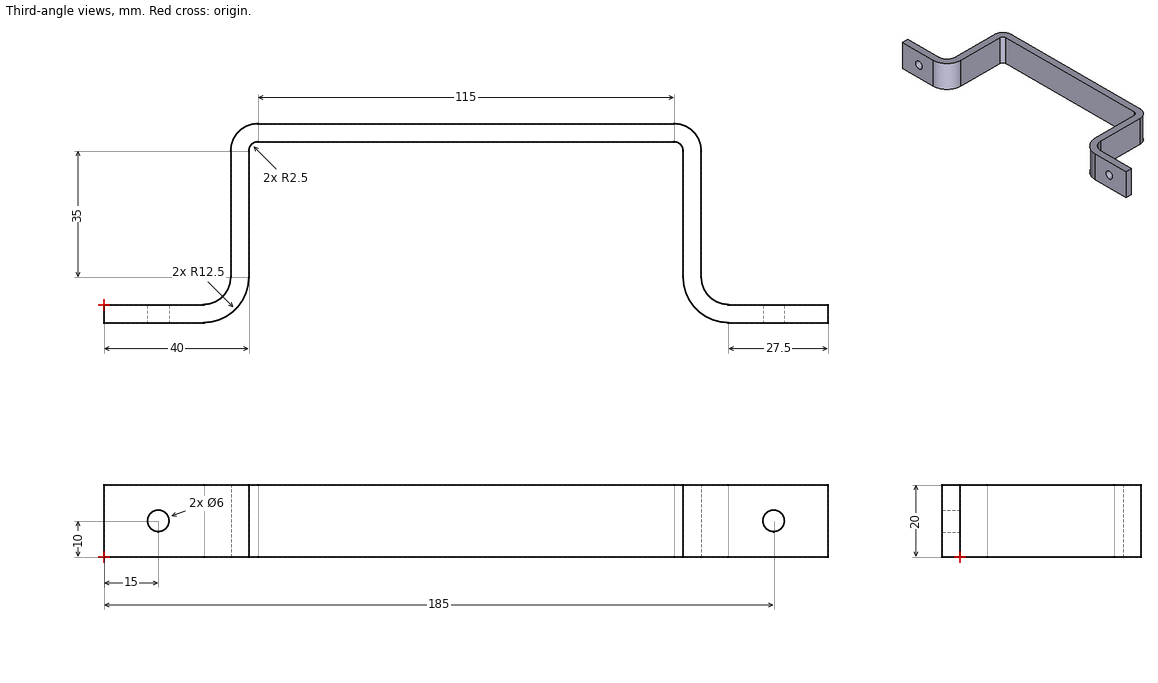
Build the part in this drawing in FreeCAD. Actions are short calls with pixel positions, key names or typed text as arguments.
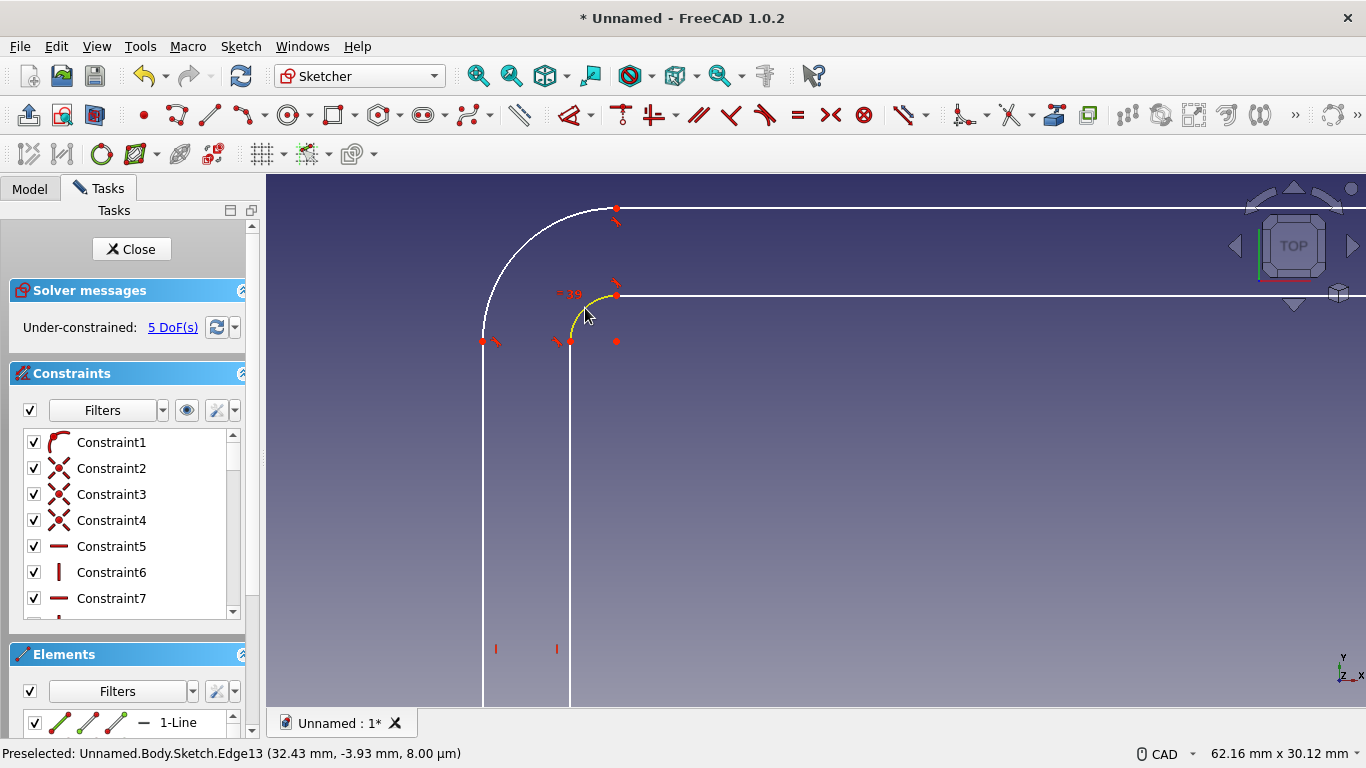
click(584, 309)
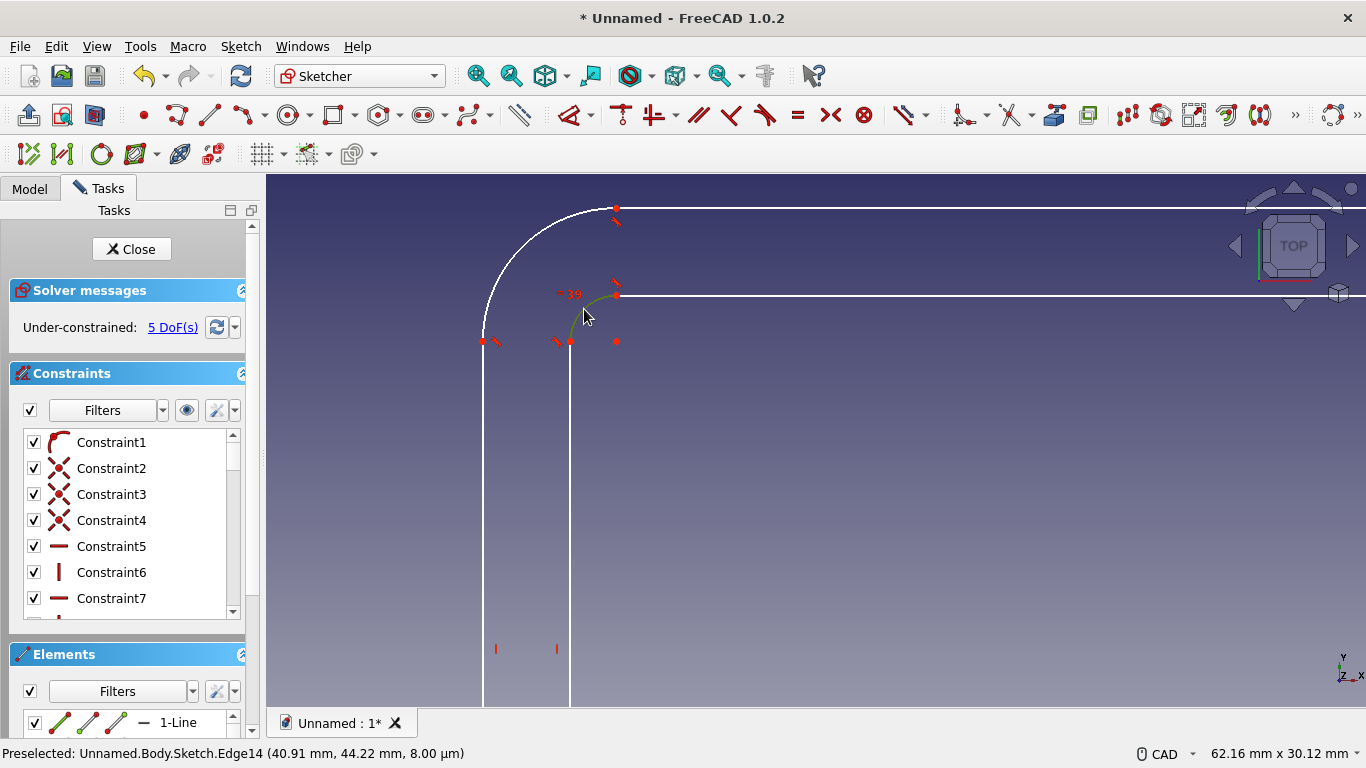
key(k)
key(r)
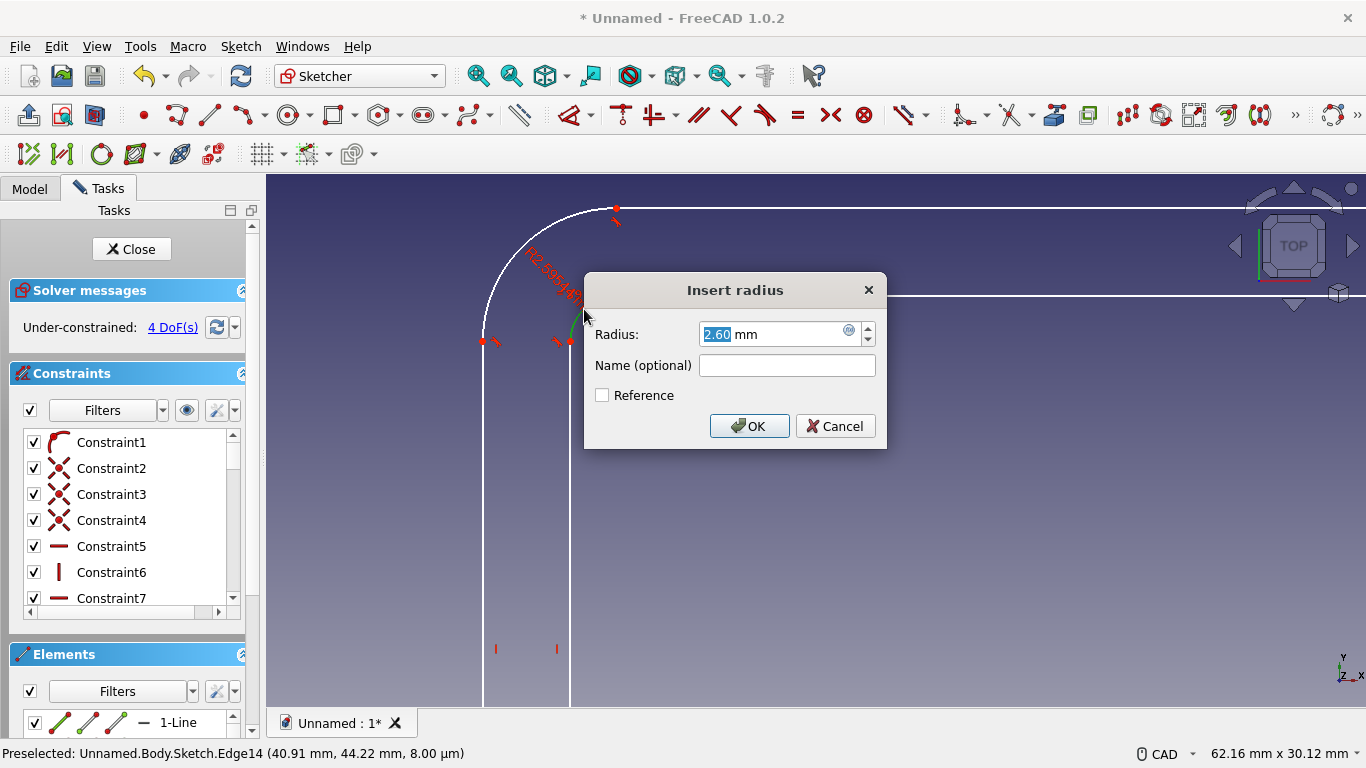
text(2.5)
key(Return)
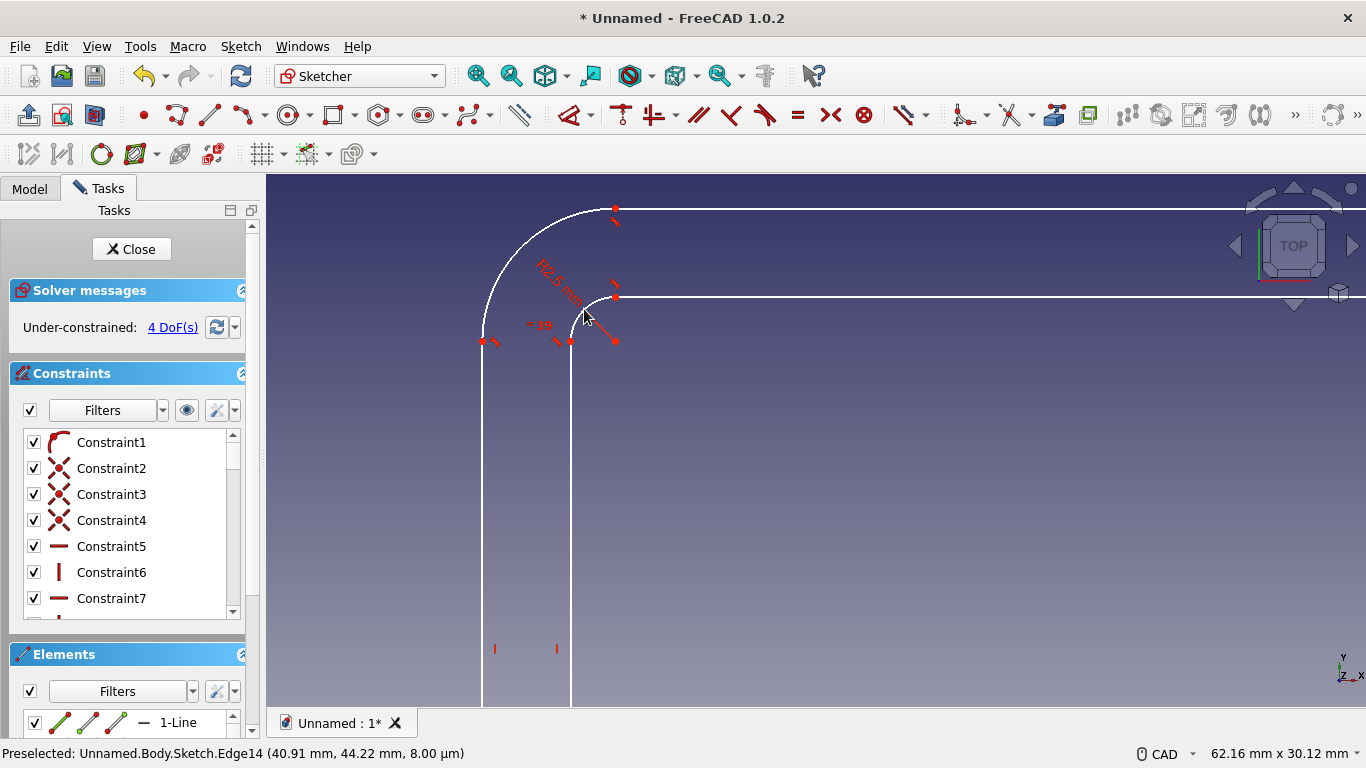
scroll(572, 391, down, 9)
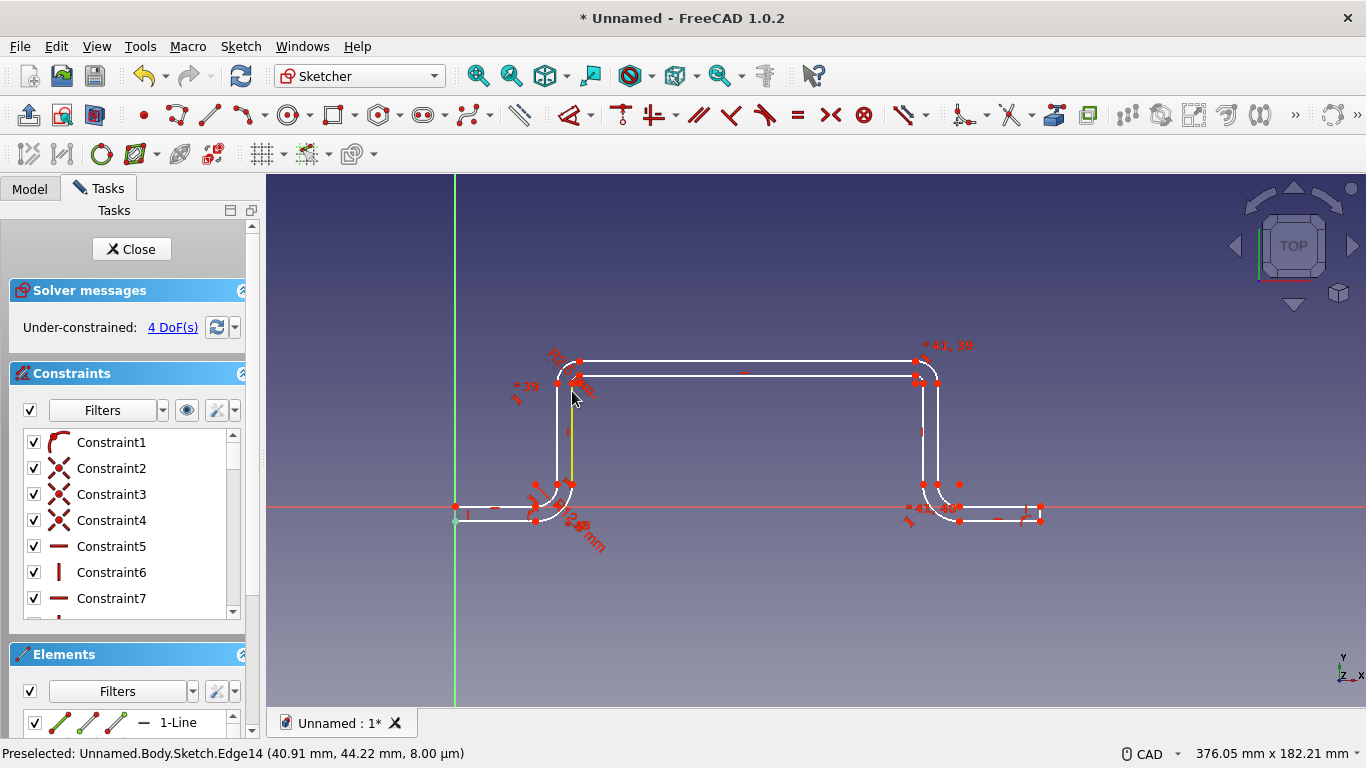
click(572, 414)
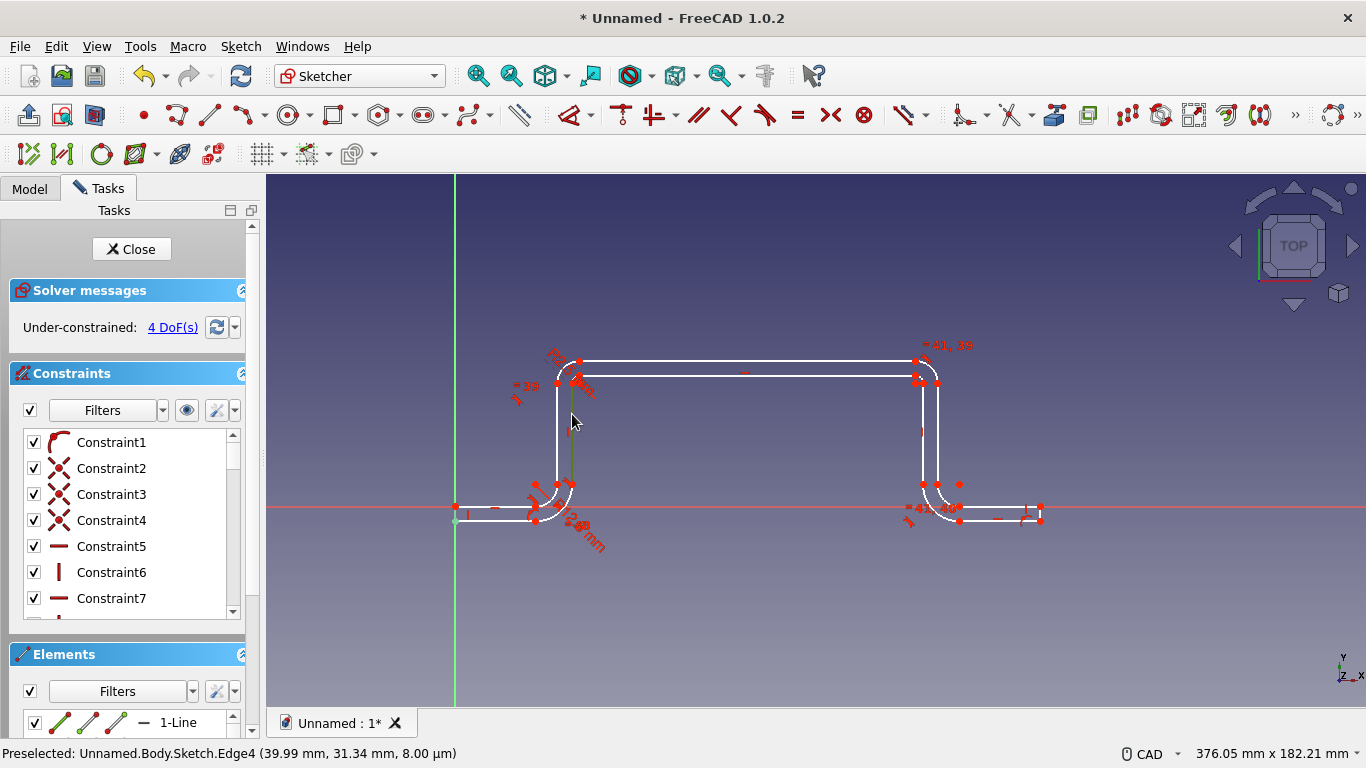
click(590, 116)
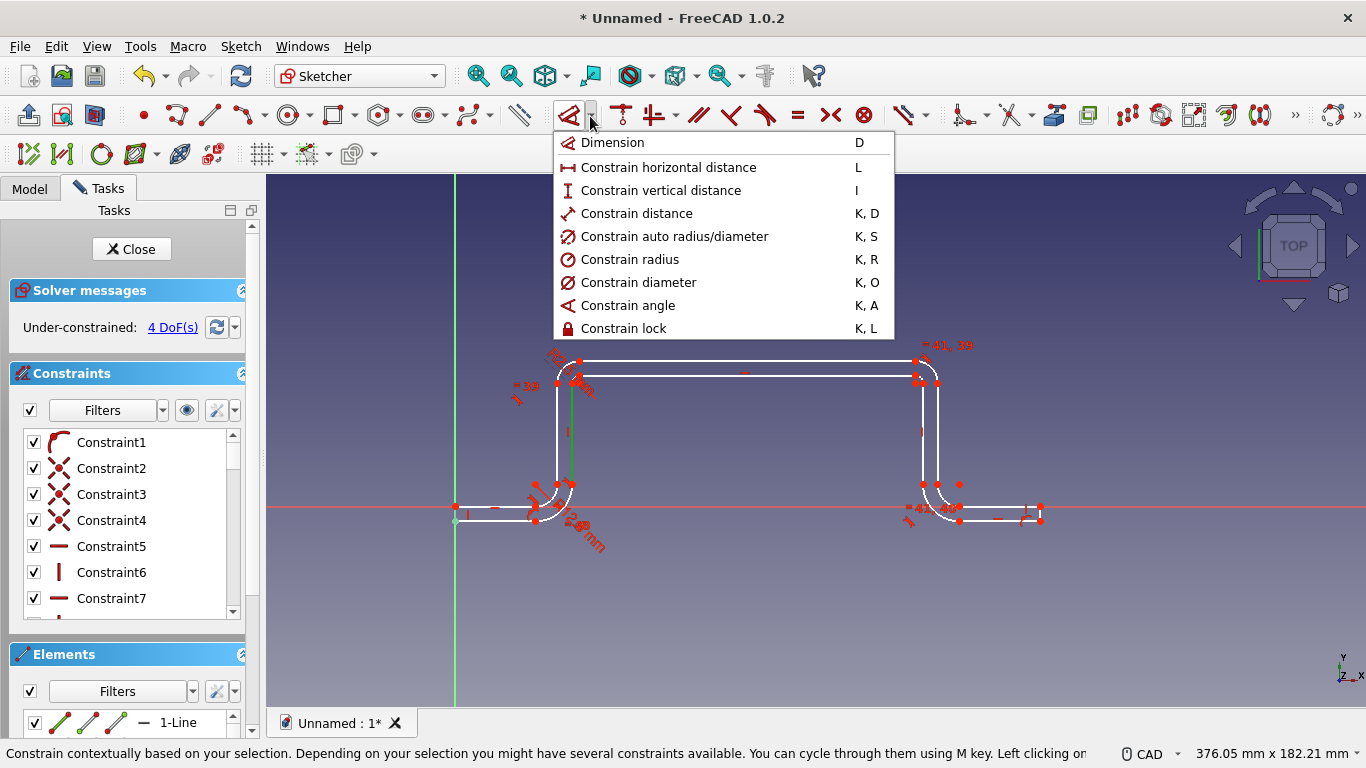
click(724, 190)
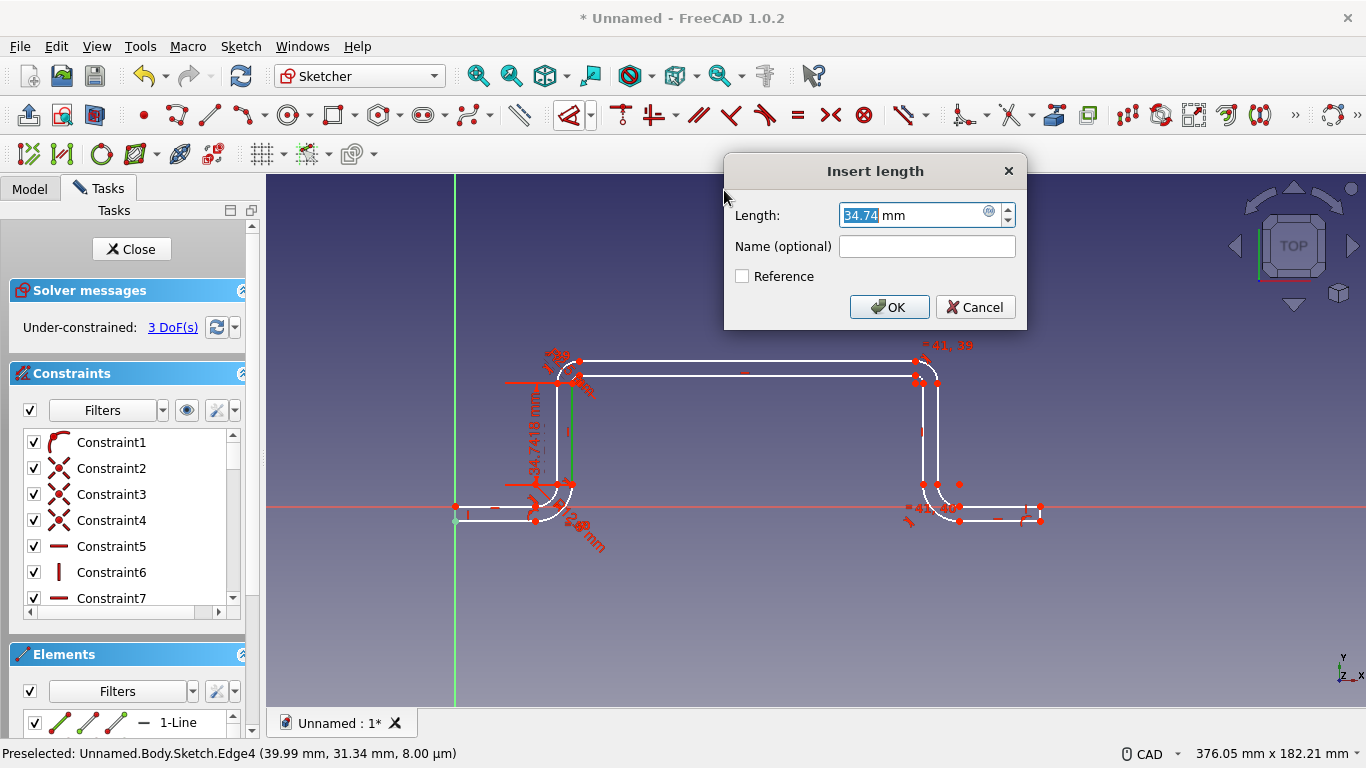
text(35)
key(Return)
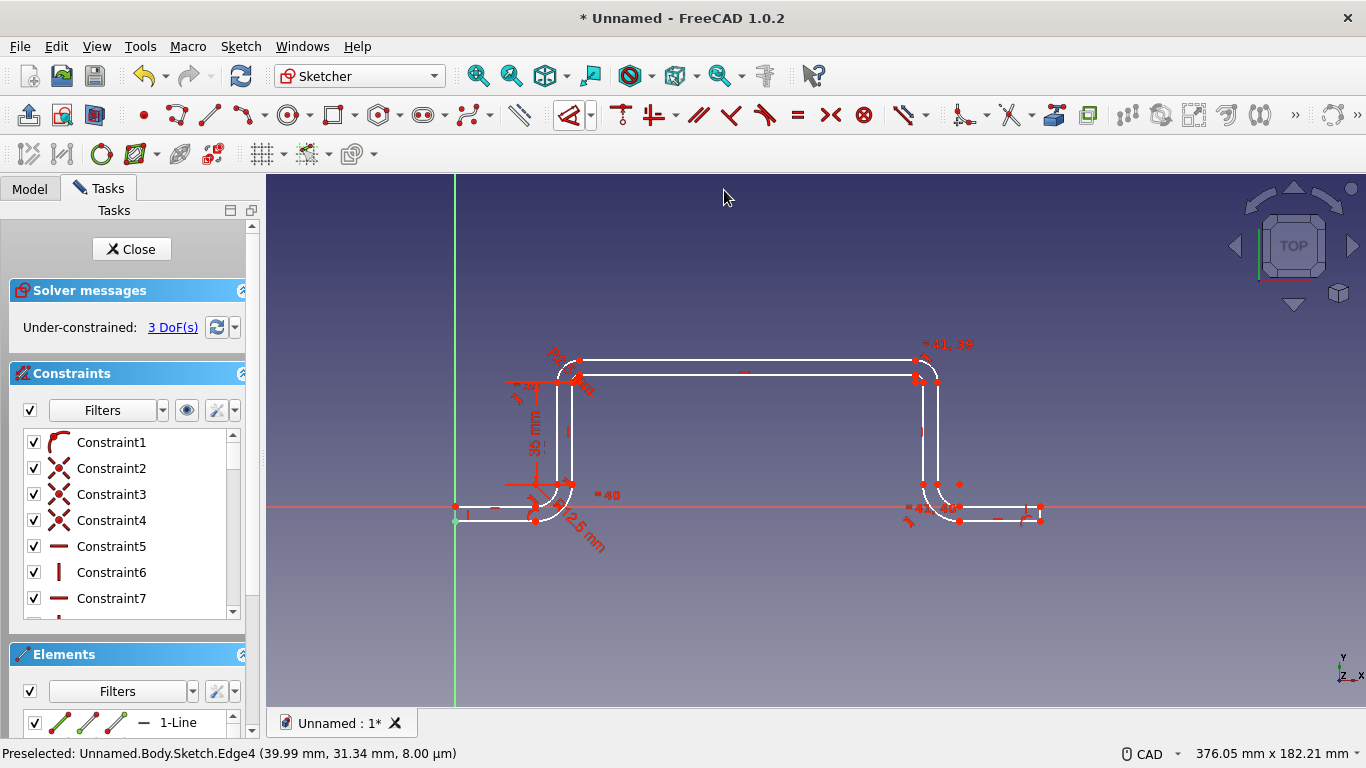
click(680, 375)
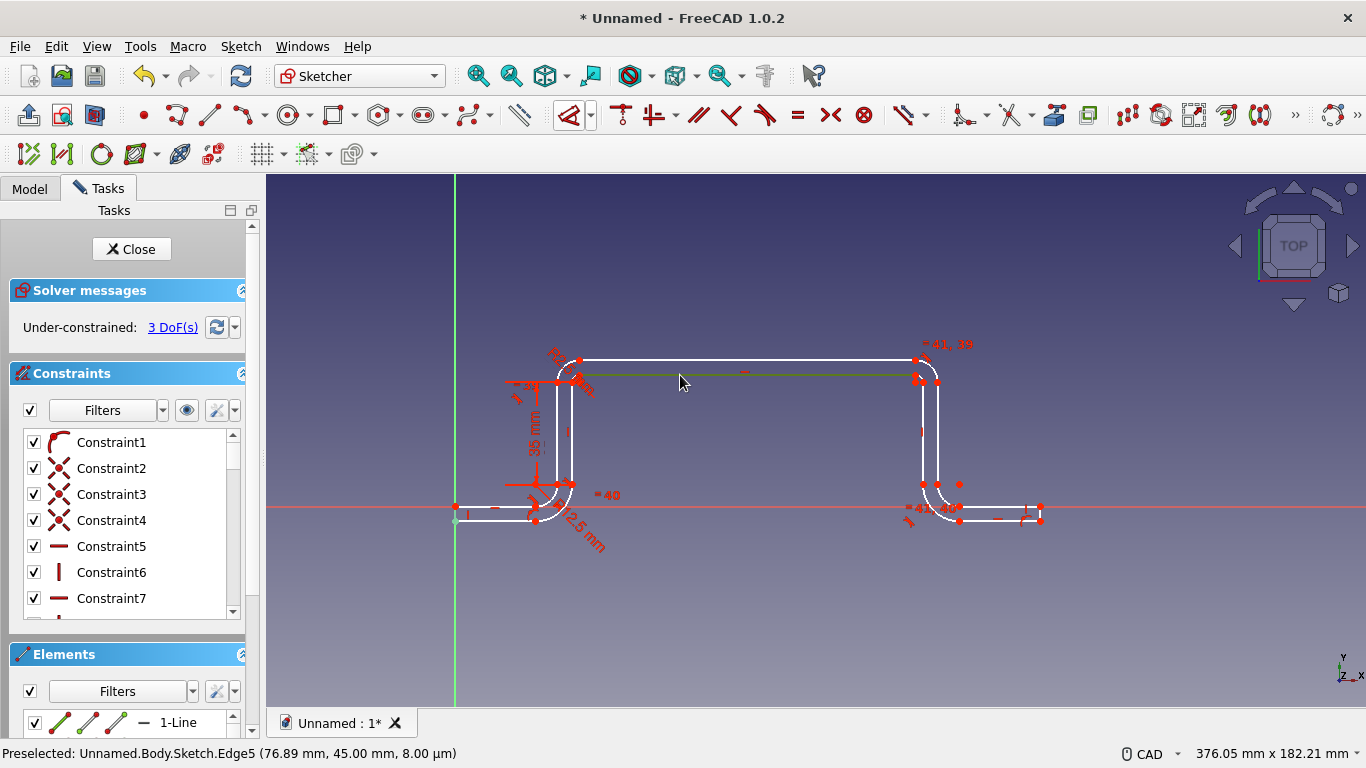
key(l)